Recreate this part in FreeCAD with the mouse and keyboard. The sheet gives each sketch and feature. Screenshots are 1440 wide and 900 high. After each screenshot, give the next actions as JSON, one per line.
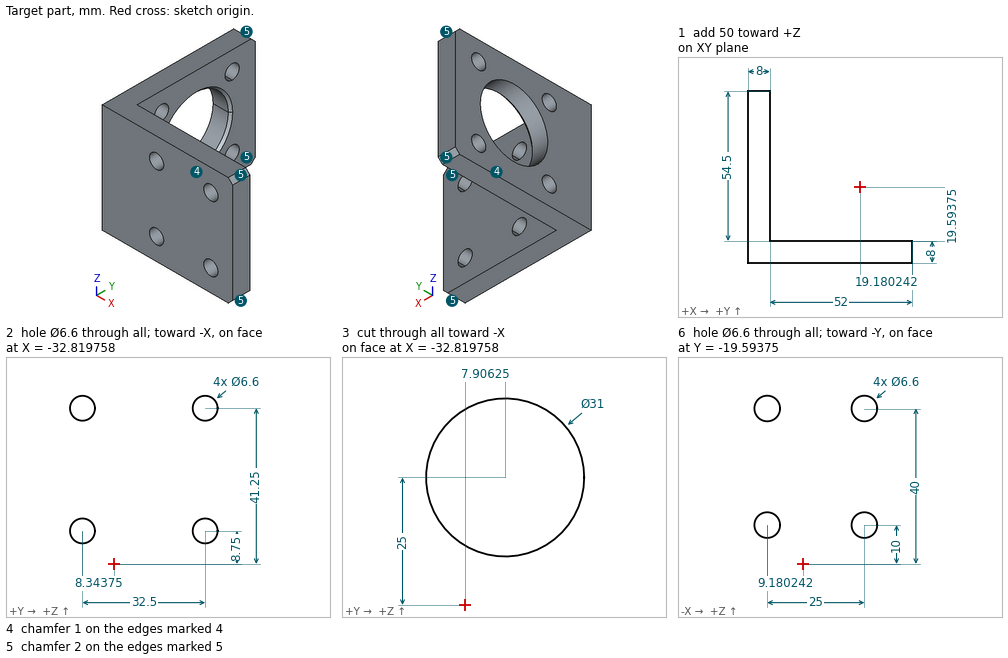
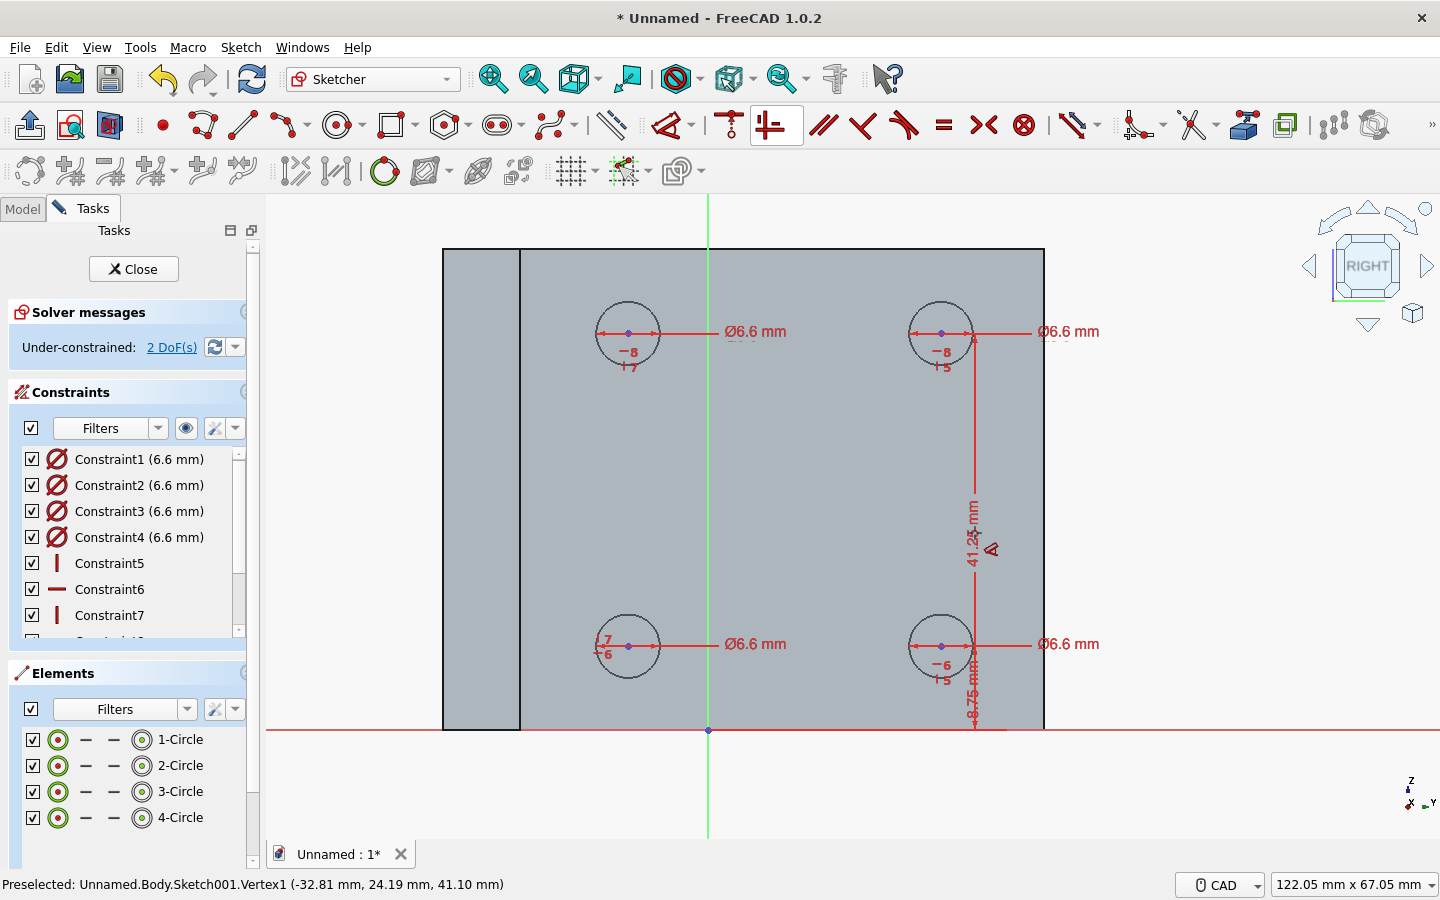
{"action": "left_click", "coordinate": [941, 646]}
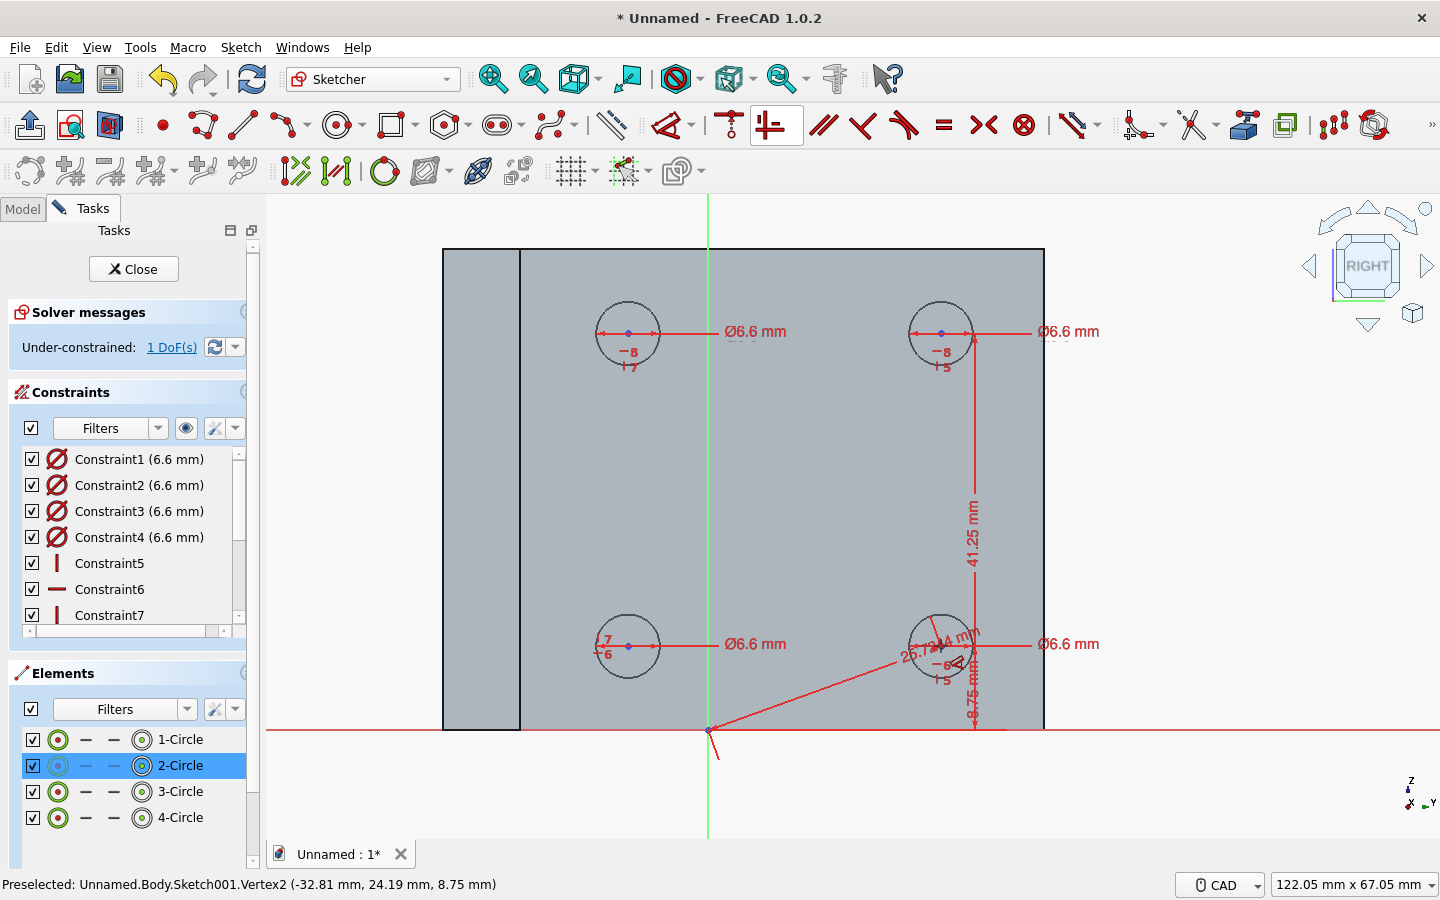
{"action": "left_click", "coordinate": [628, 646]}
{"action": "left_click", "coordinate": [785, 680]}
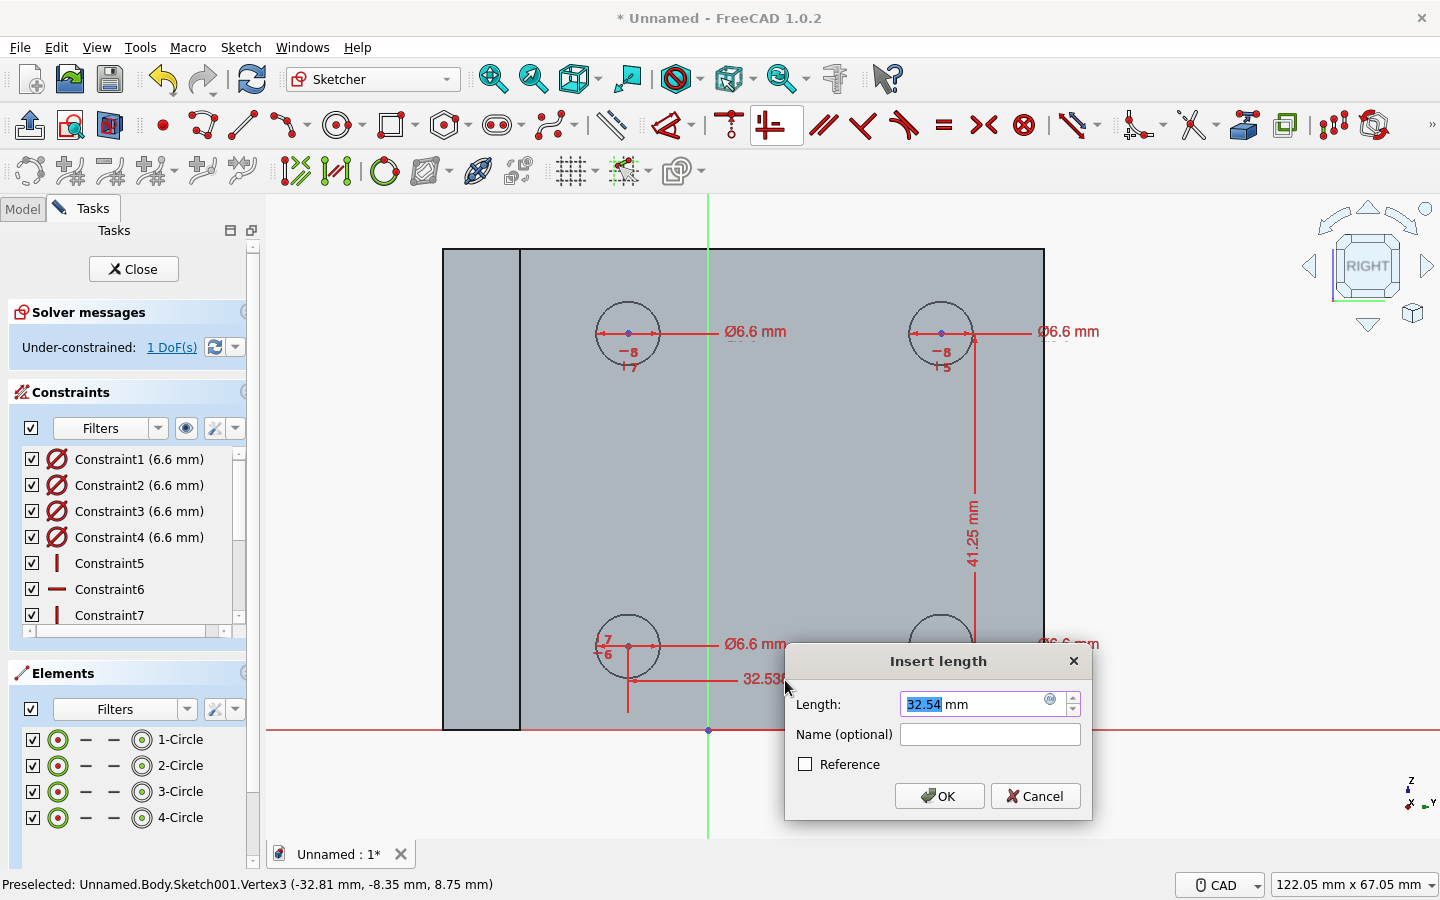
{"action": "type", "text": "32.5"}
{"action": "key", "text": "Return"}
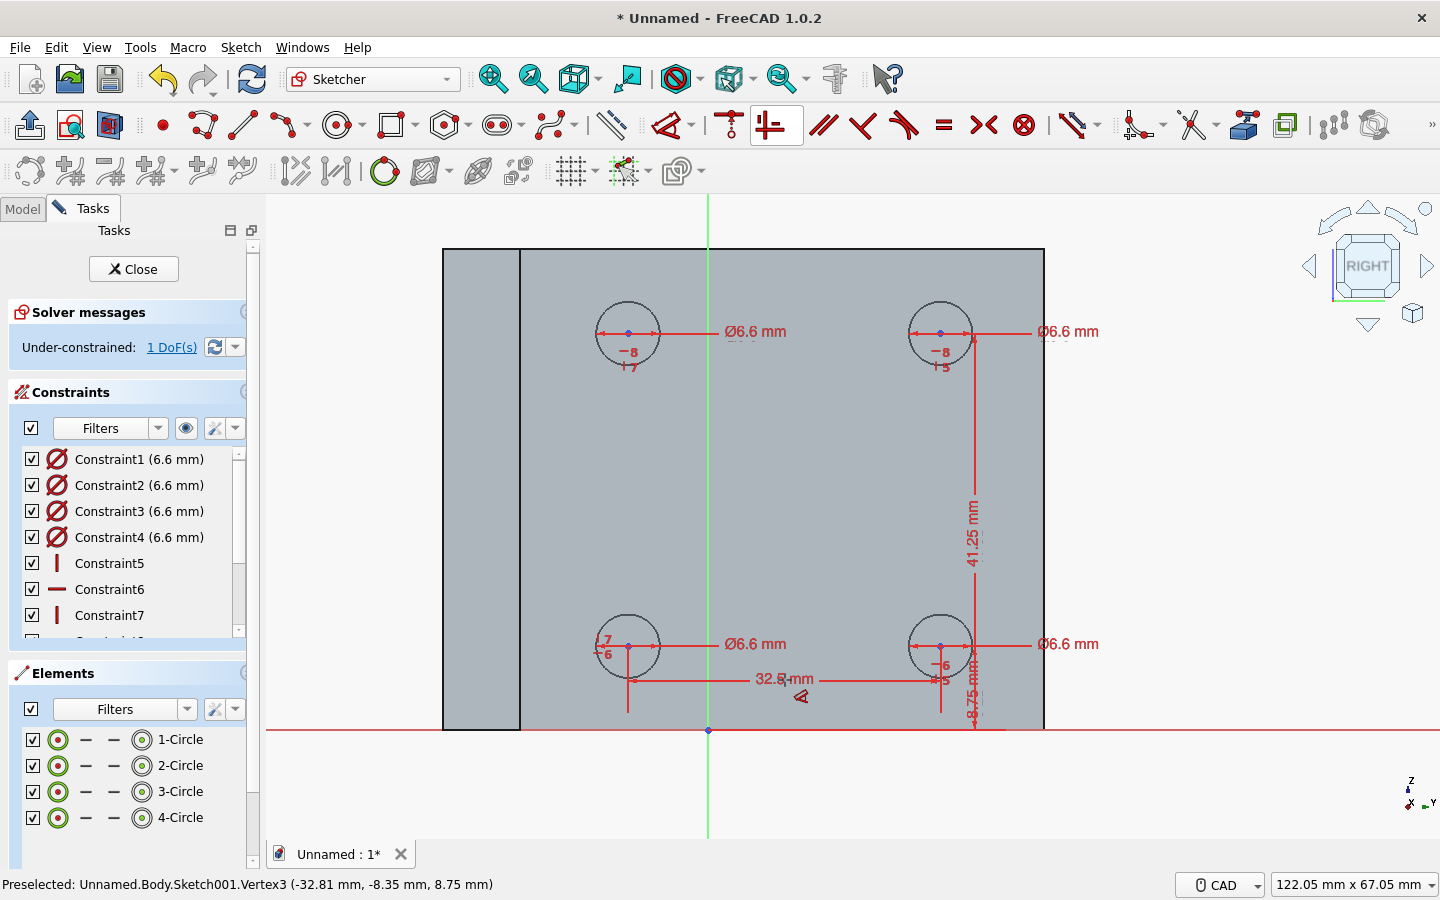
{"action": "left_click", "coordinate": [628, 646]}
{"action": "left_click", "coordinate": [668, 764]}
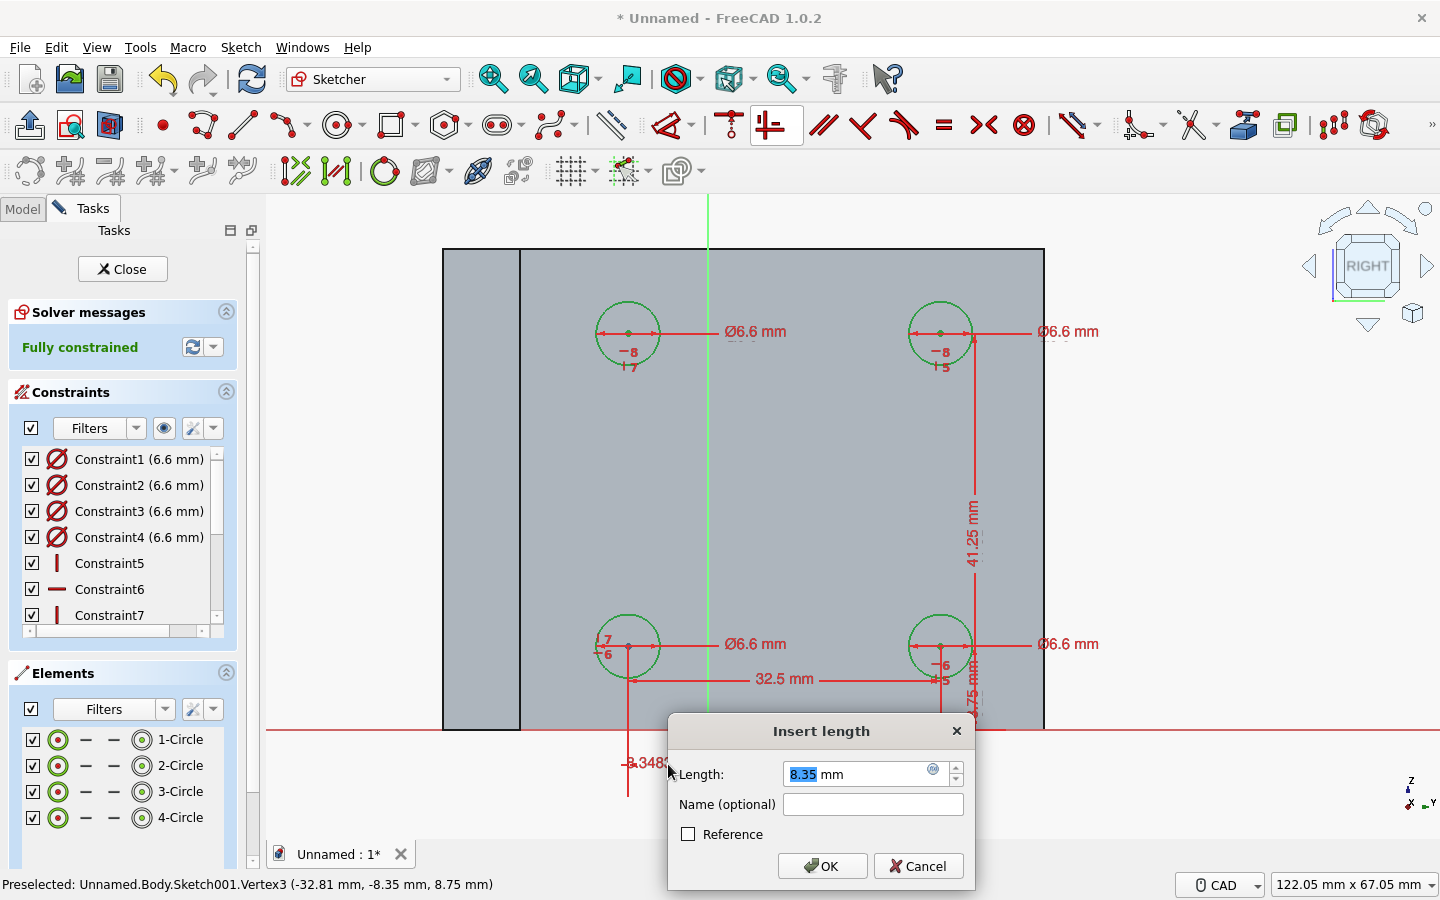
{"action": "type", "text": "8.34375"}
{"action": "key", "text": "Return"}
{"action": "key", "text": "Escape"}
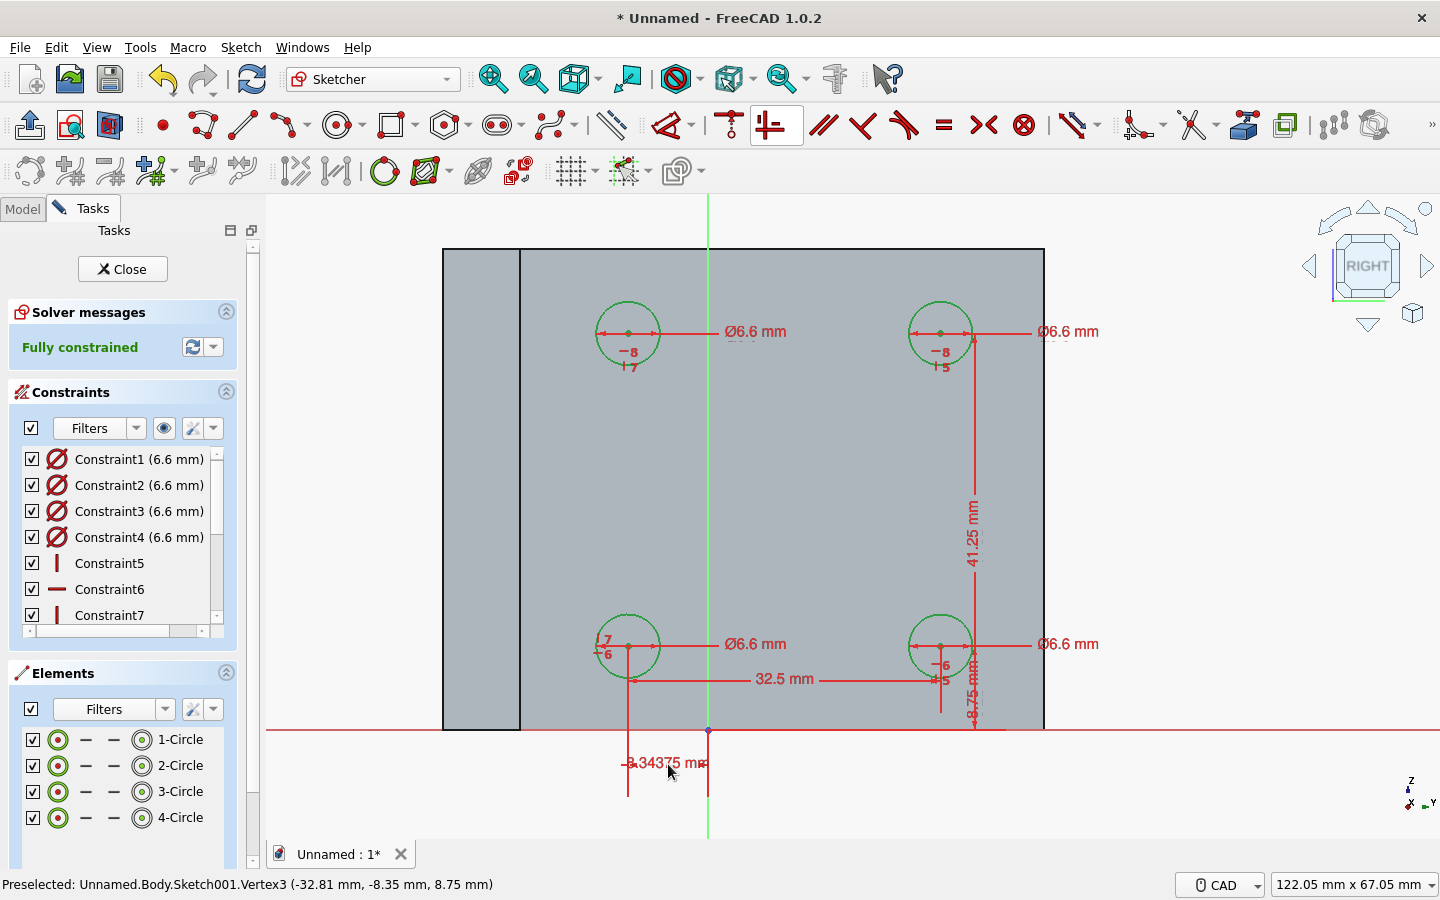
{"action": "left_click", "coordinate": [123, 269]}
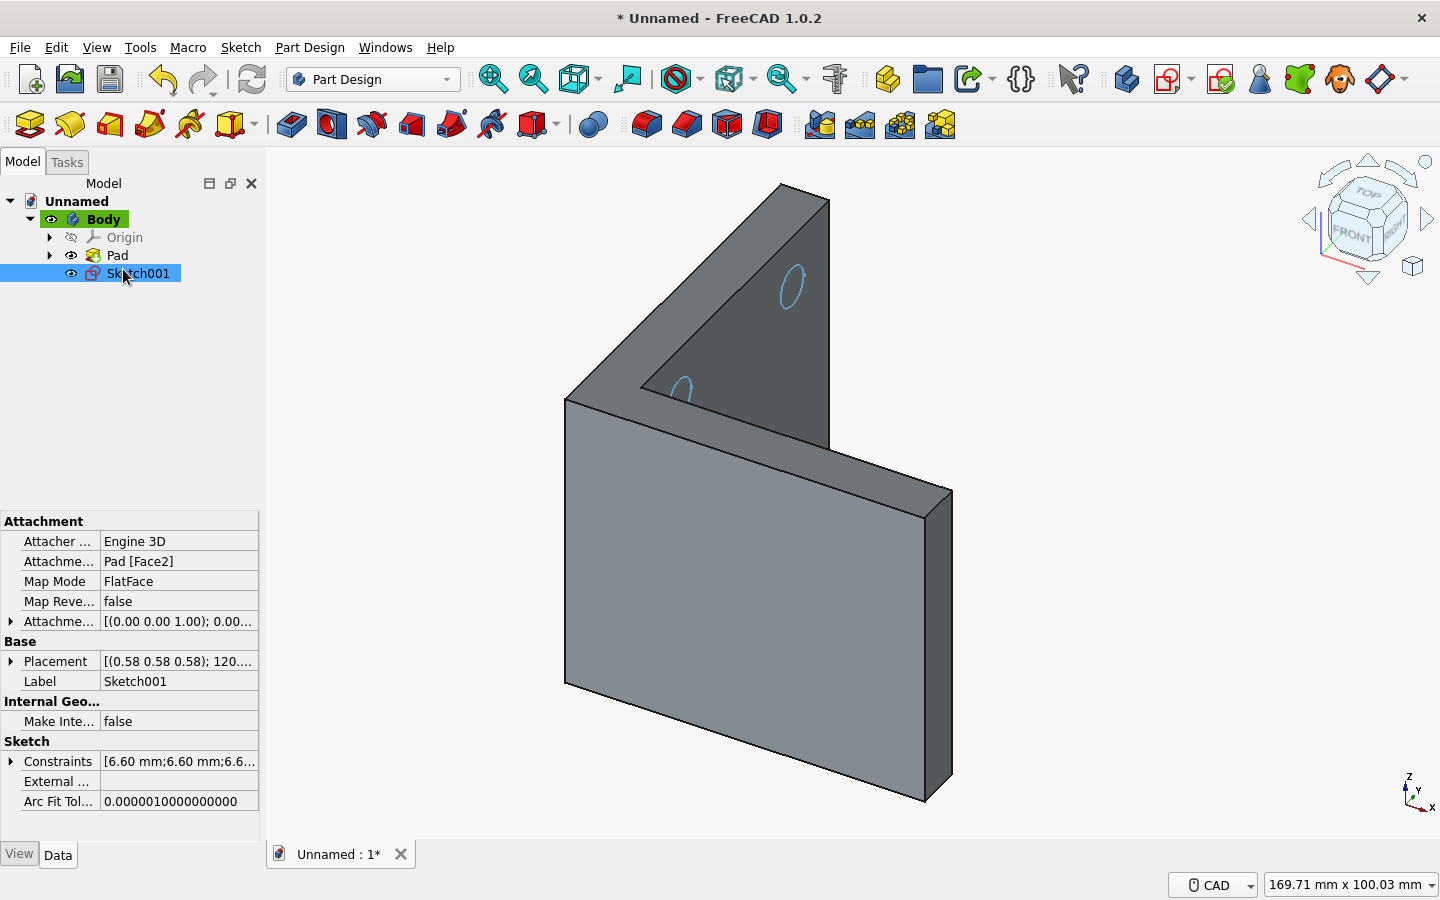
{"action": "left_click", "coordinate": [332, 124]}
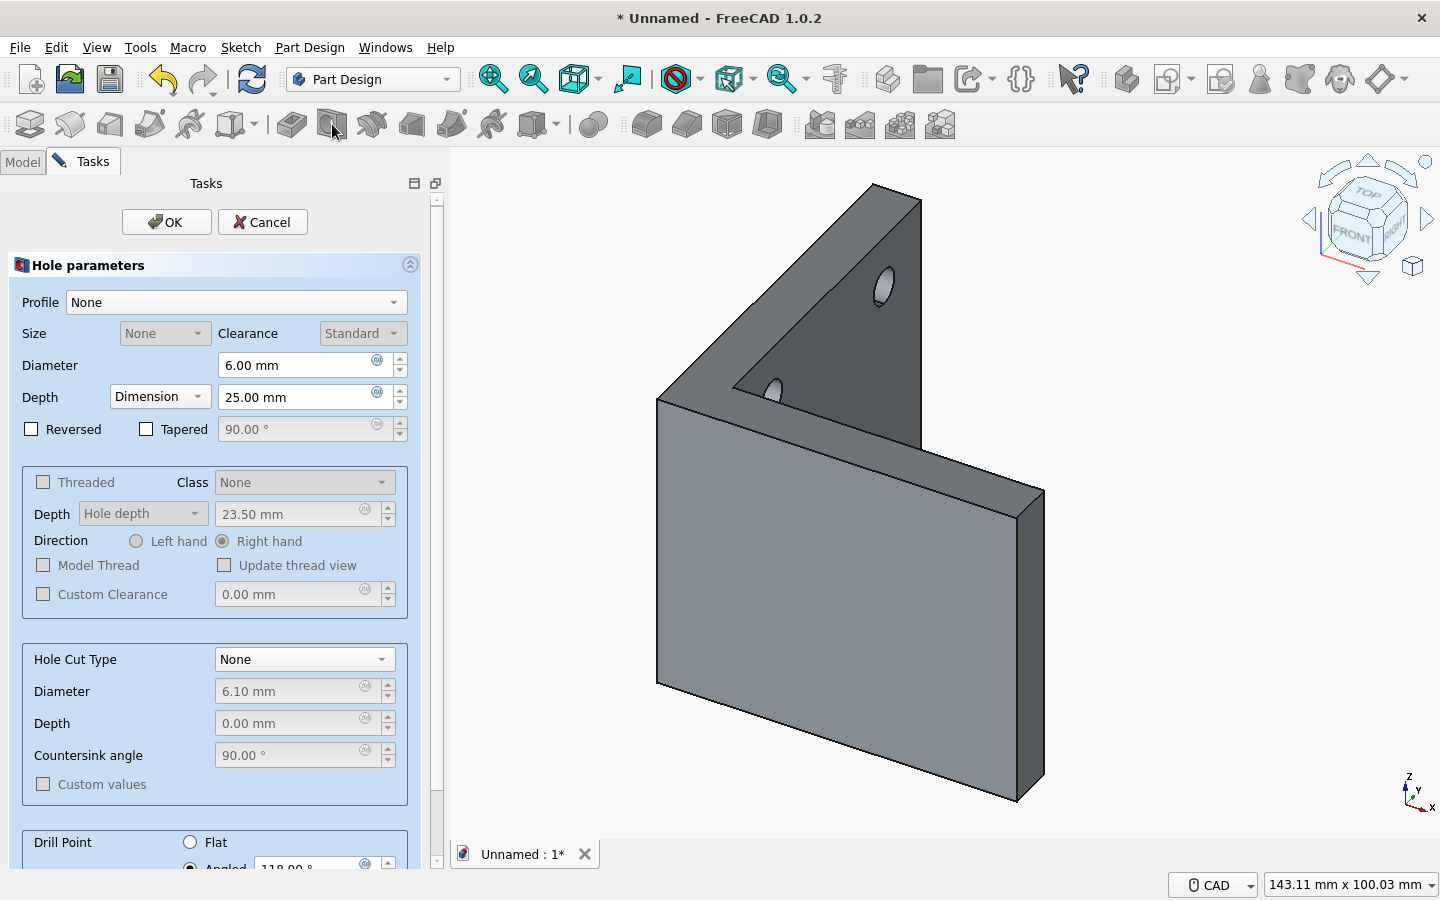
{"action": "triple_click", "coordinate": [305, 365]}